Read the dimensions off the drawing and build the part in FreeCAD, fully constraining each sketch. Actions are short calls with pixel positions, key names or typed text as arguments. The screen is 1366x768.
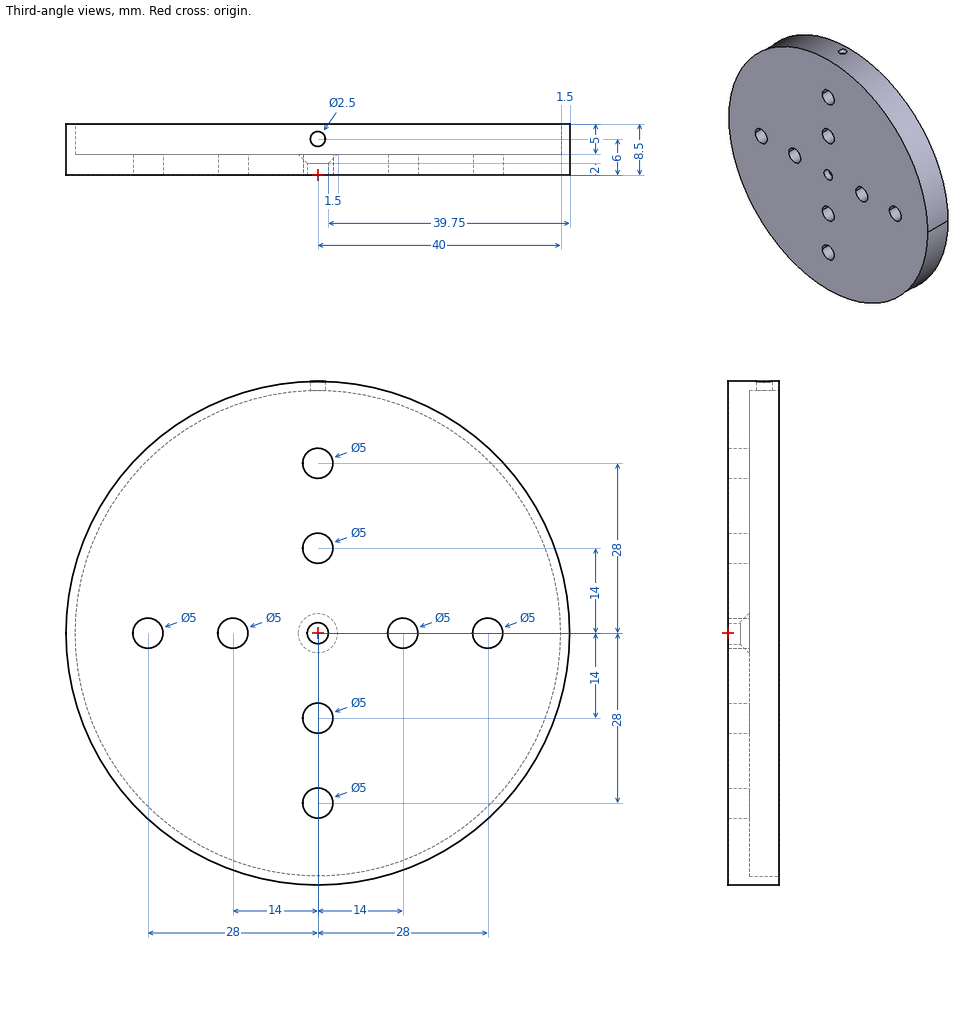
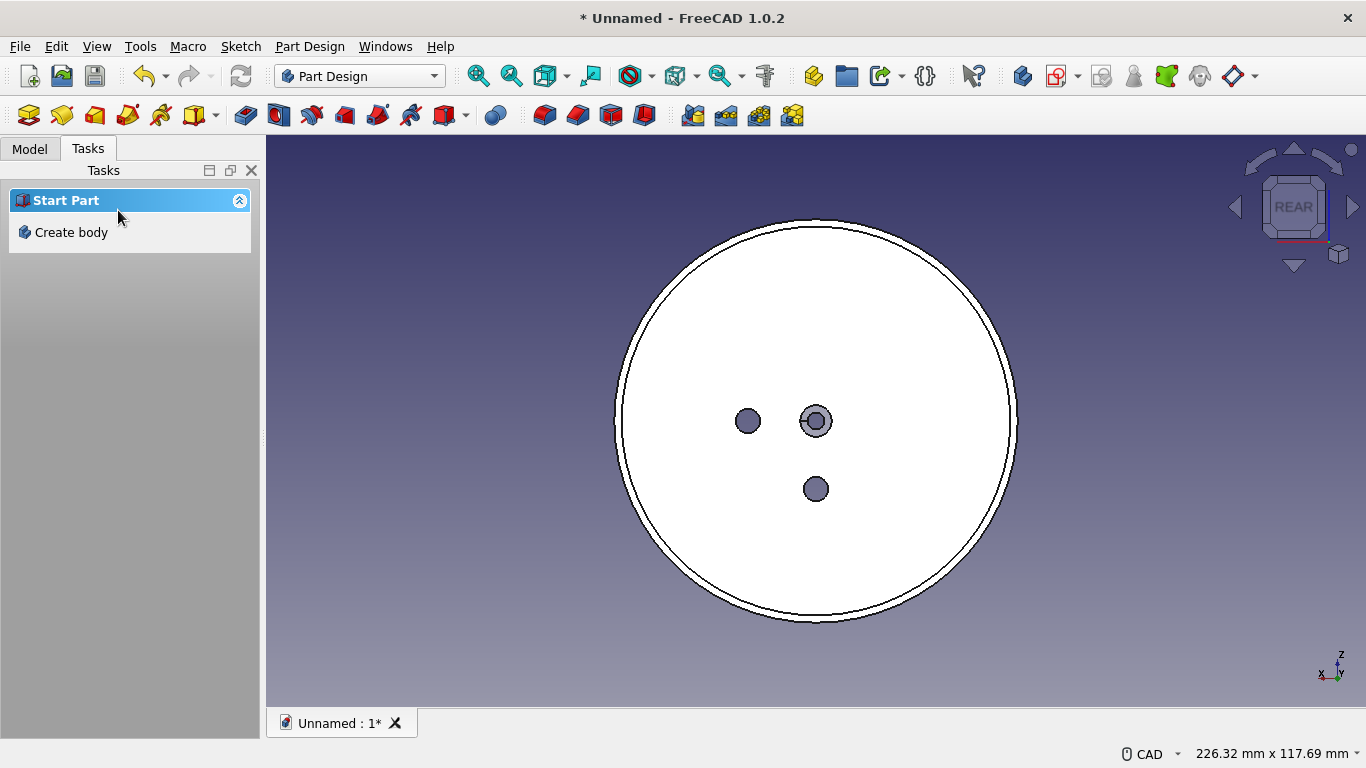
click(816, 309)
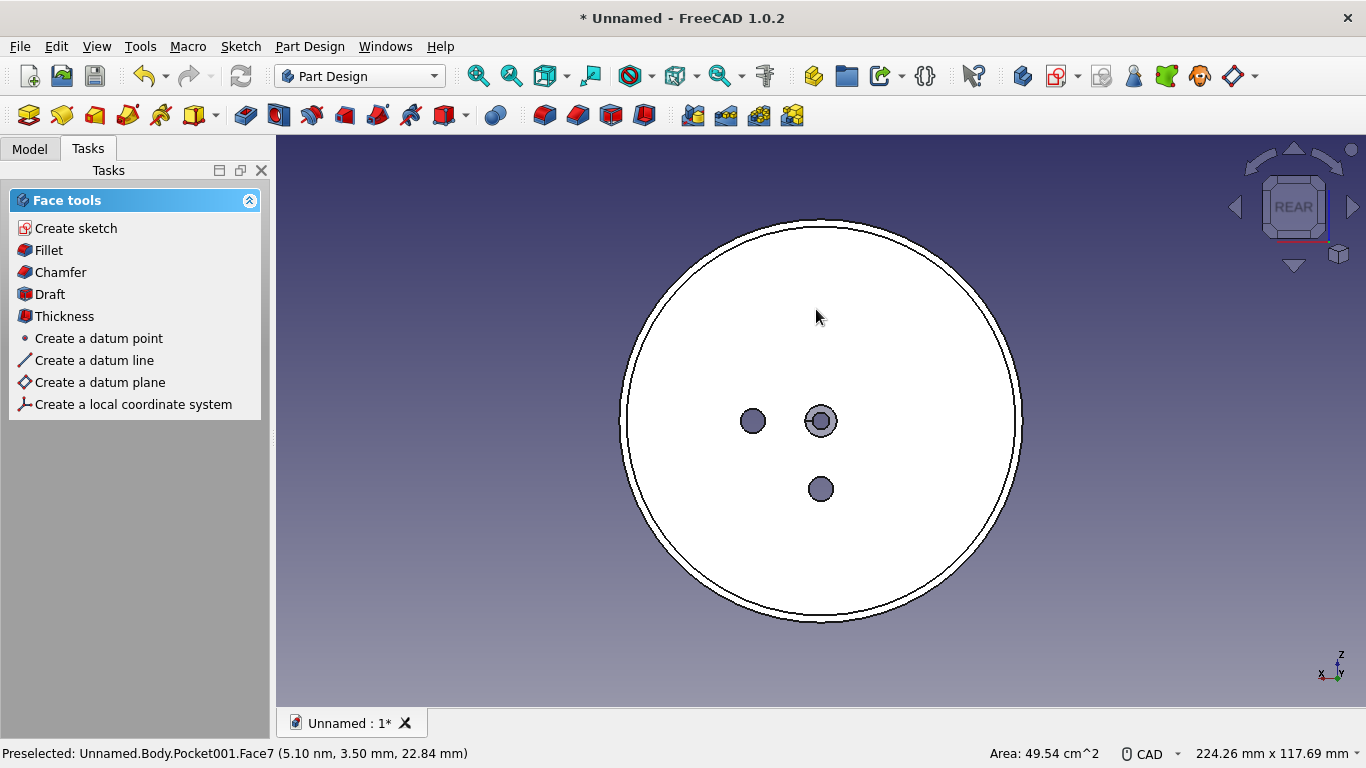
click(1056, 76)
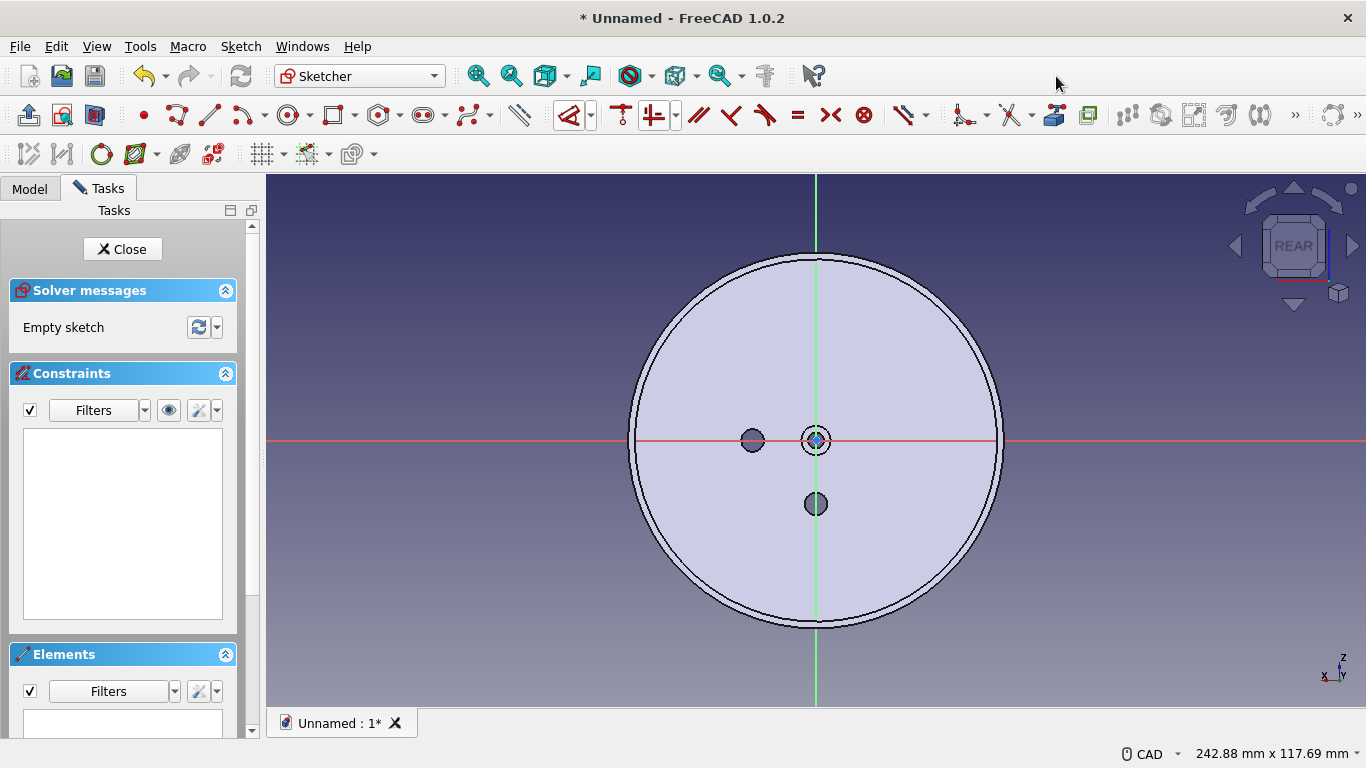
click(95, 116)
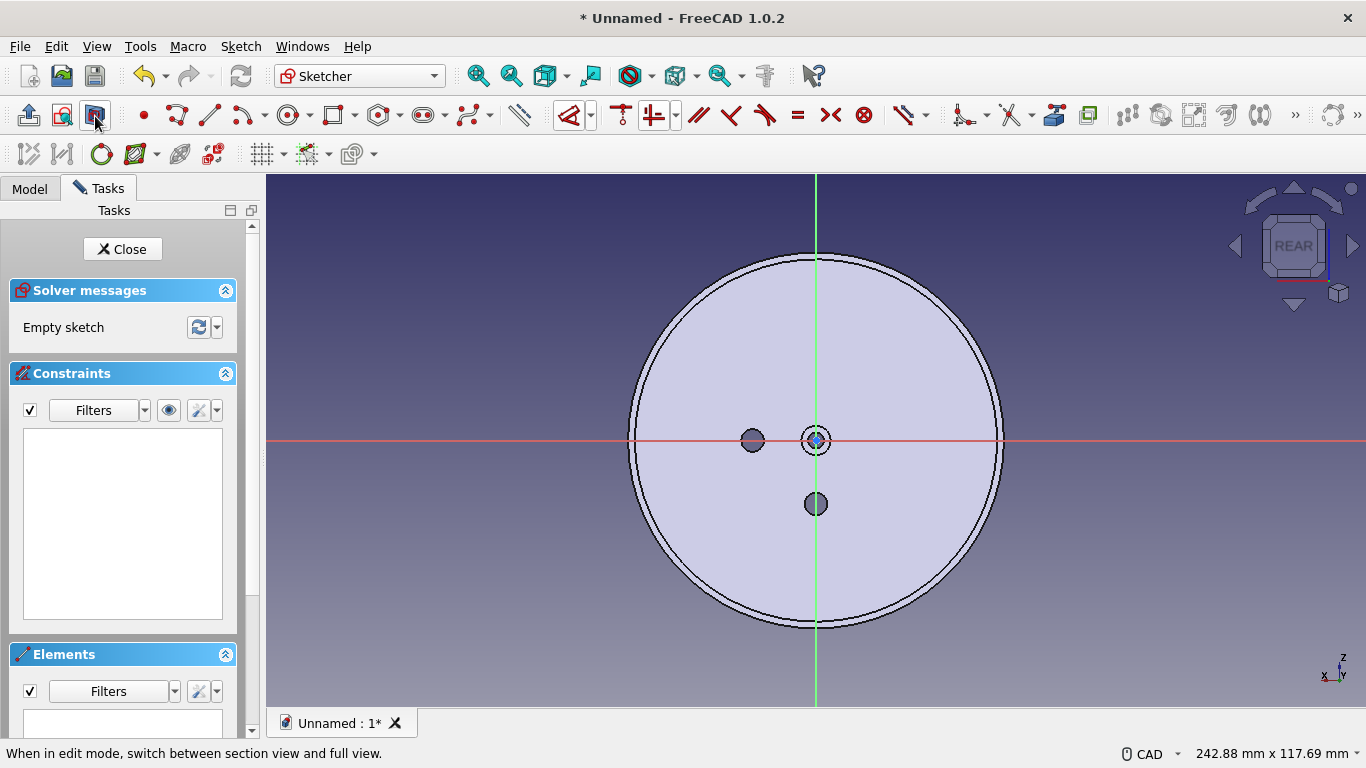
scroll(821, 577, up, 13)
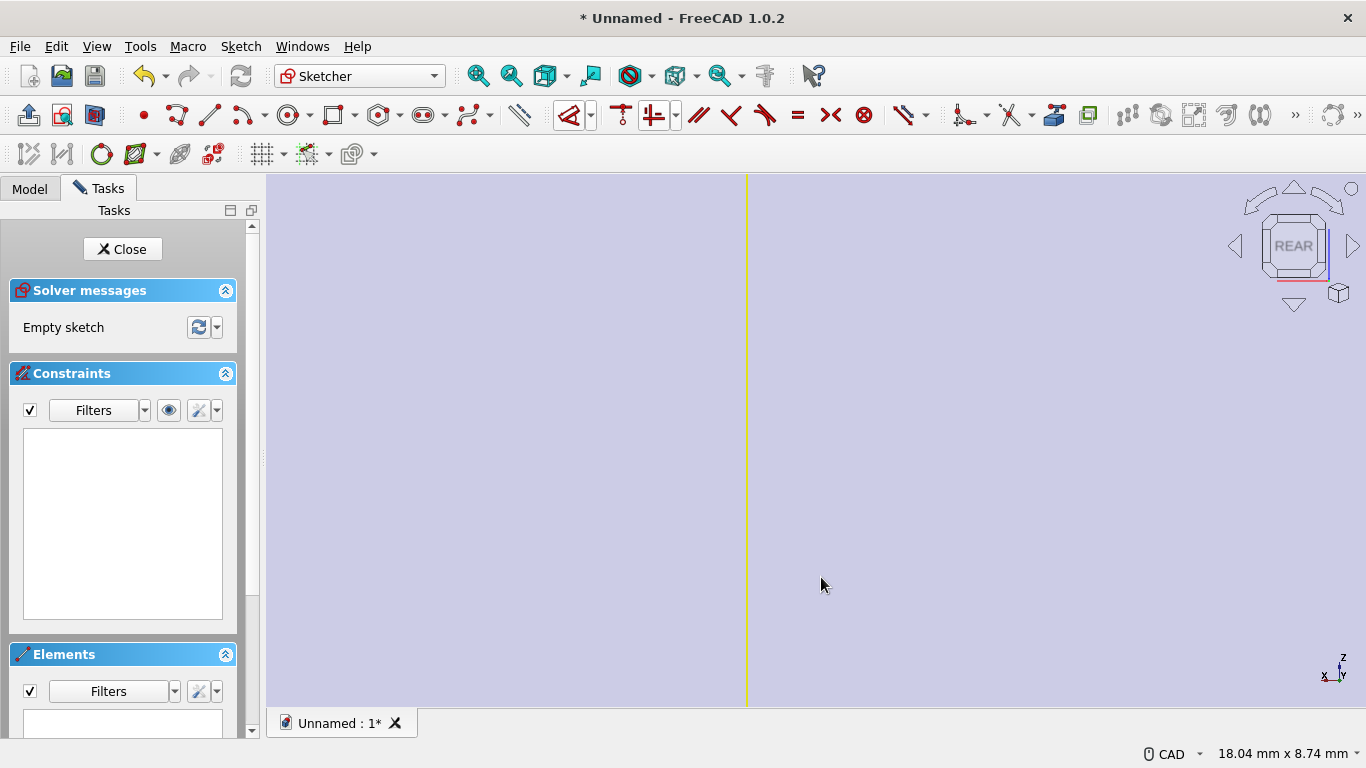
click(288, 116)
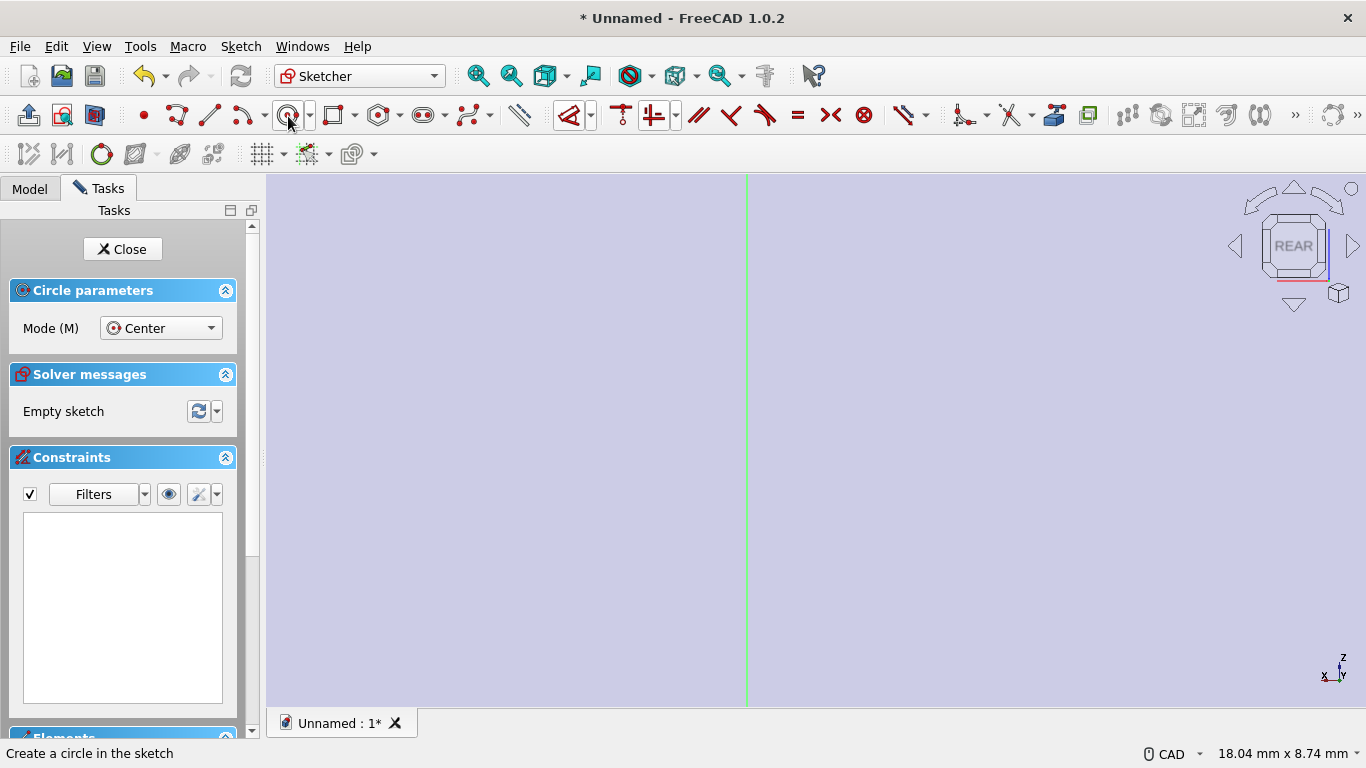
click(747, 437)
click(855, 329)
key(Escape)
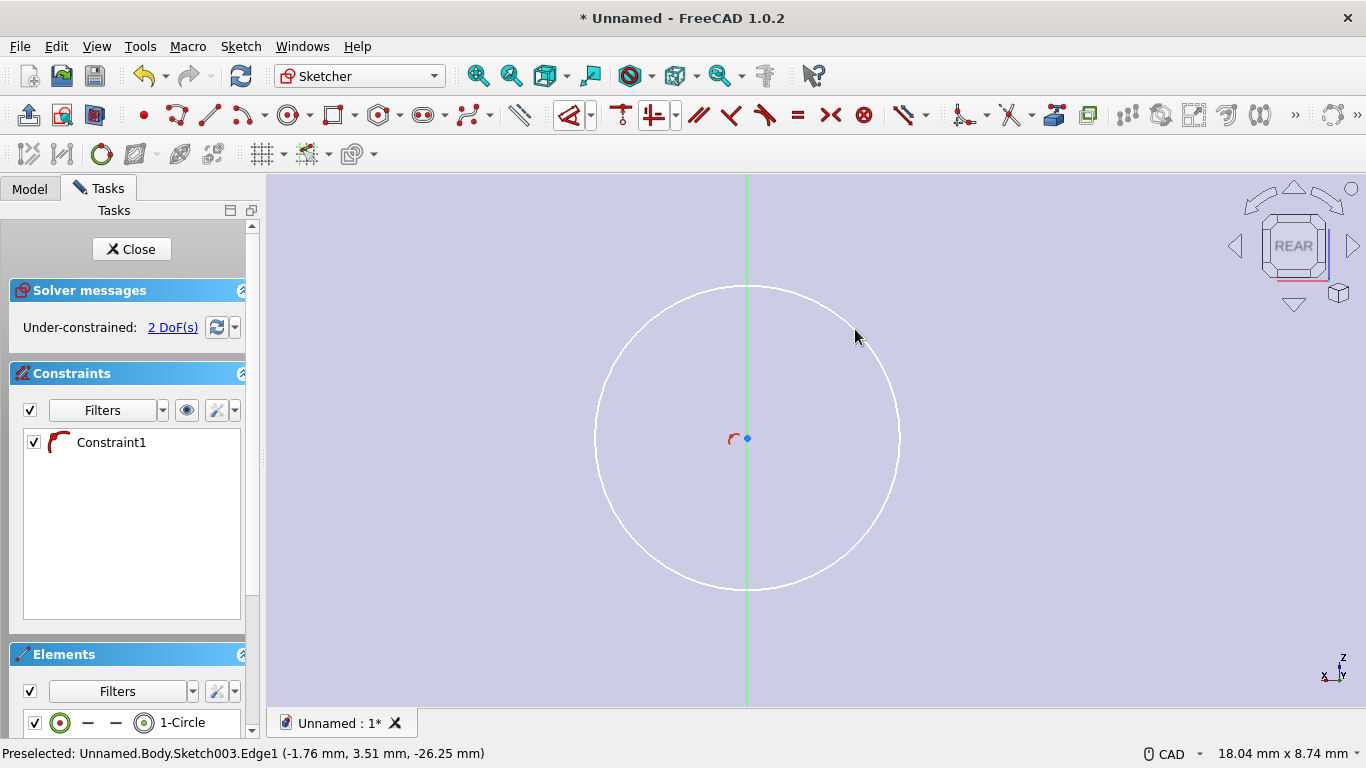
click(855, 330)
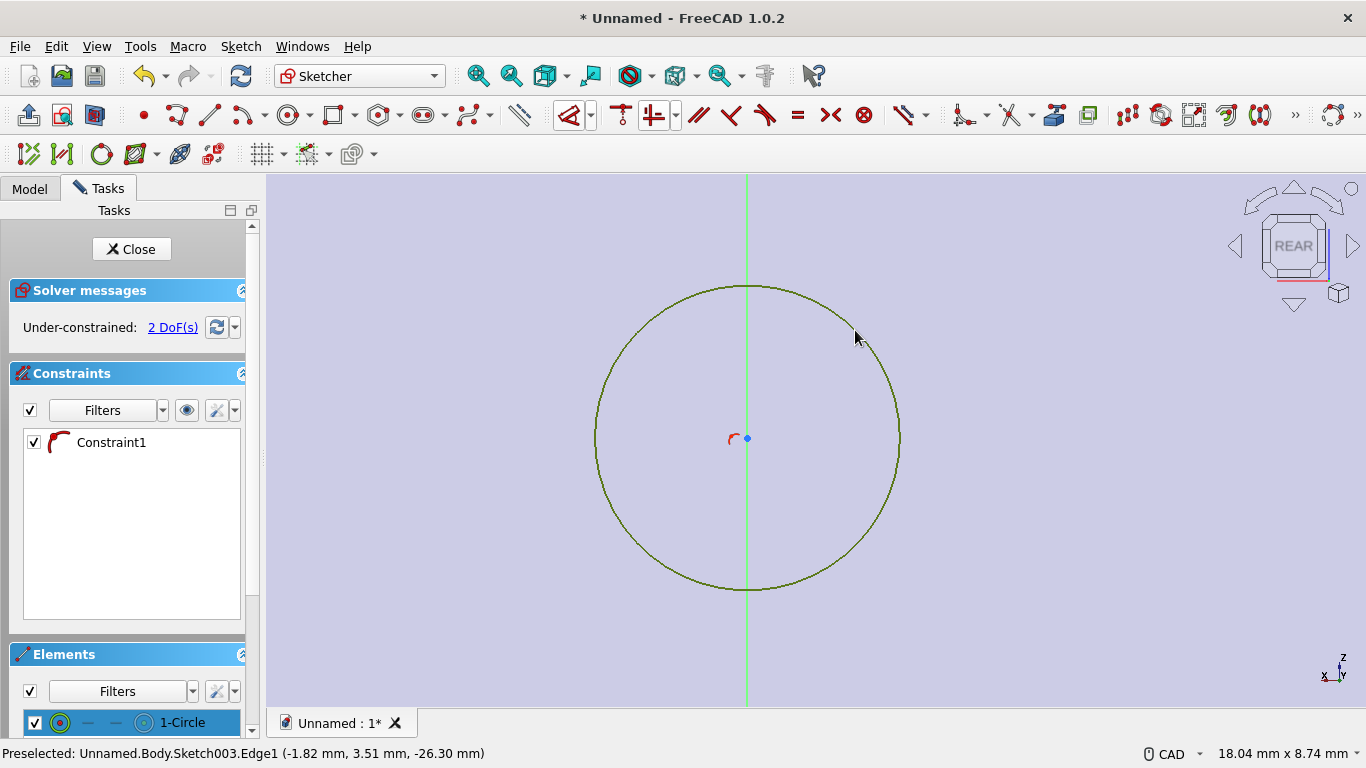
click(590, 116)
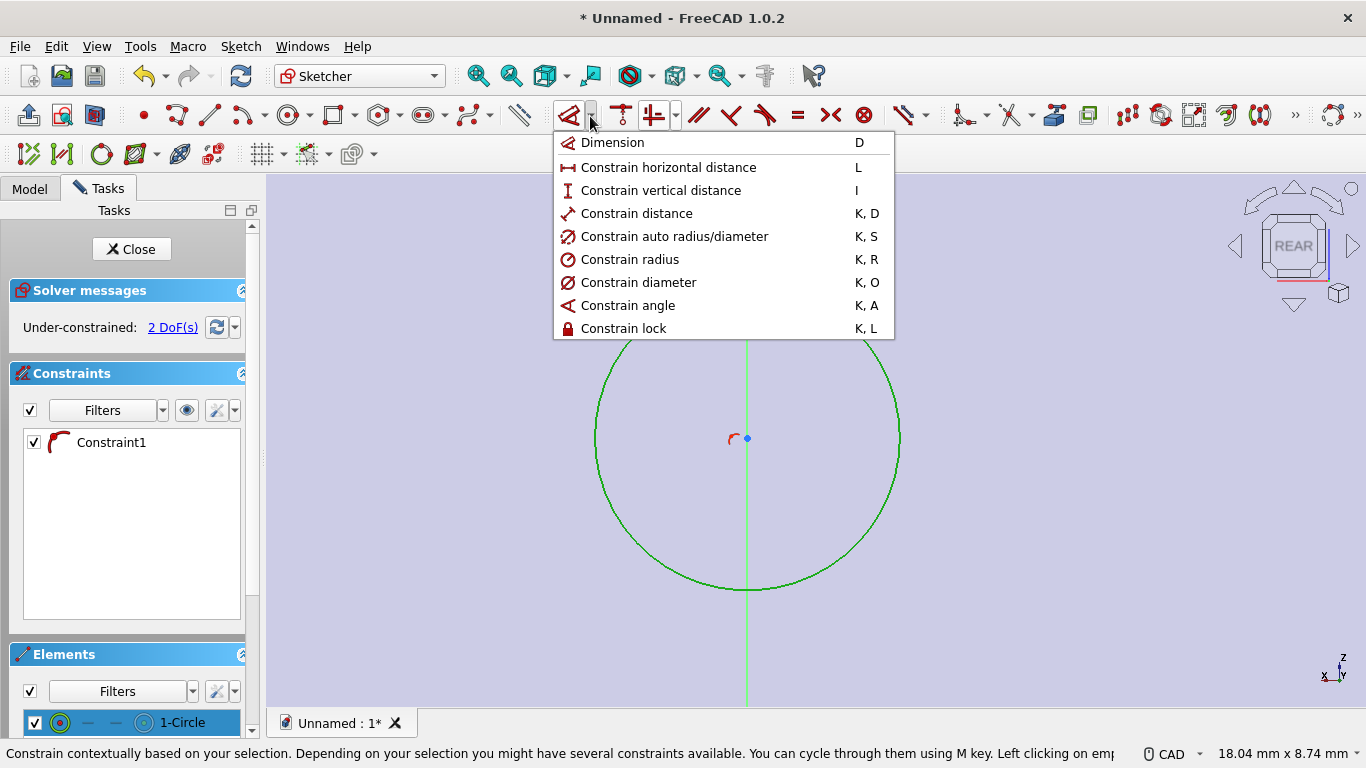
click(724, 282)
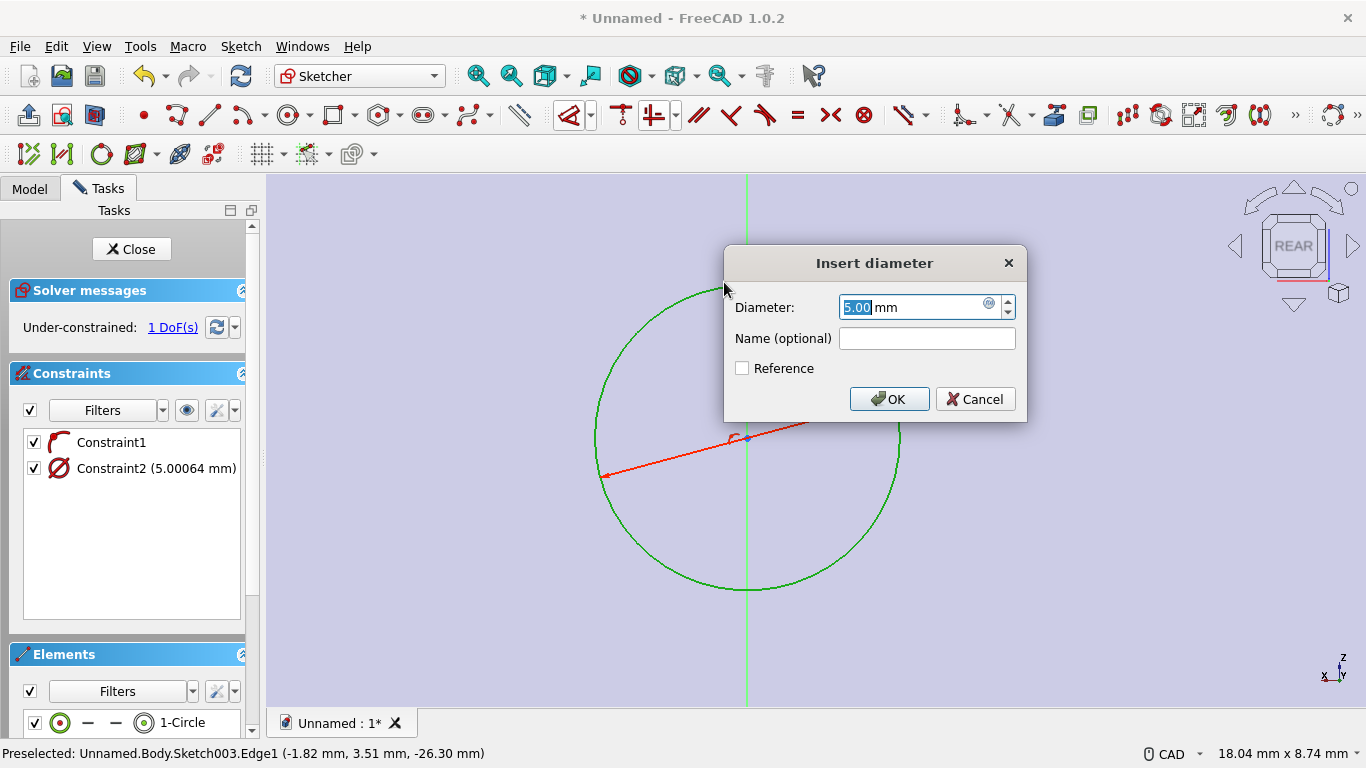
text(5)
key(Return)